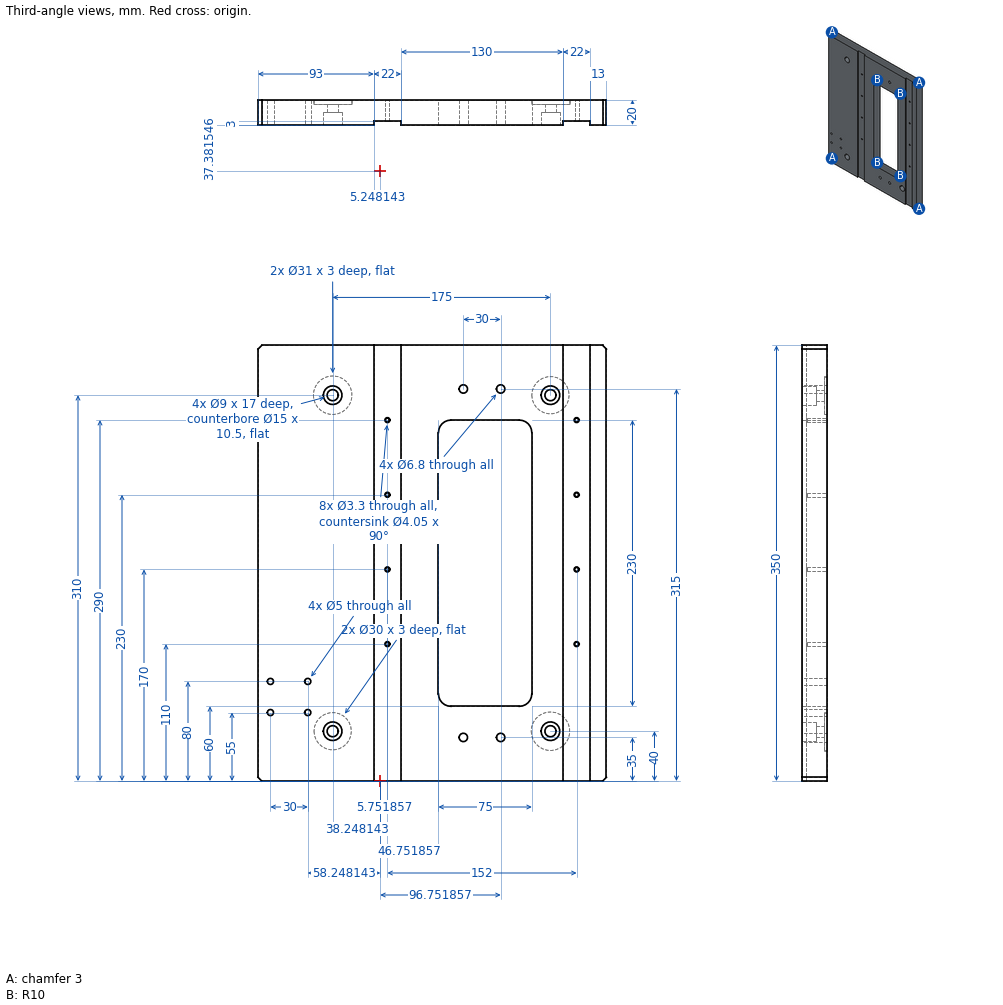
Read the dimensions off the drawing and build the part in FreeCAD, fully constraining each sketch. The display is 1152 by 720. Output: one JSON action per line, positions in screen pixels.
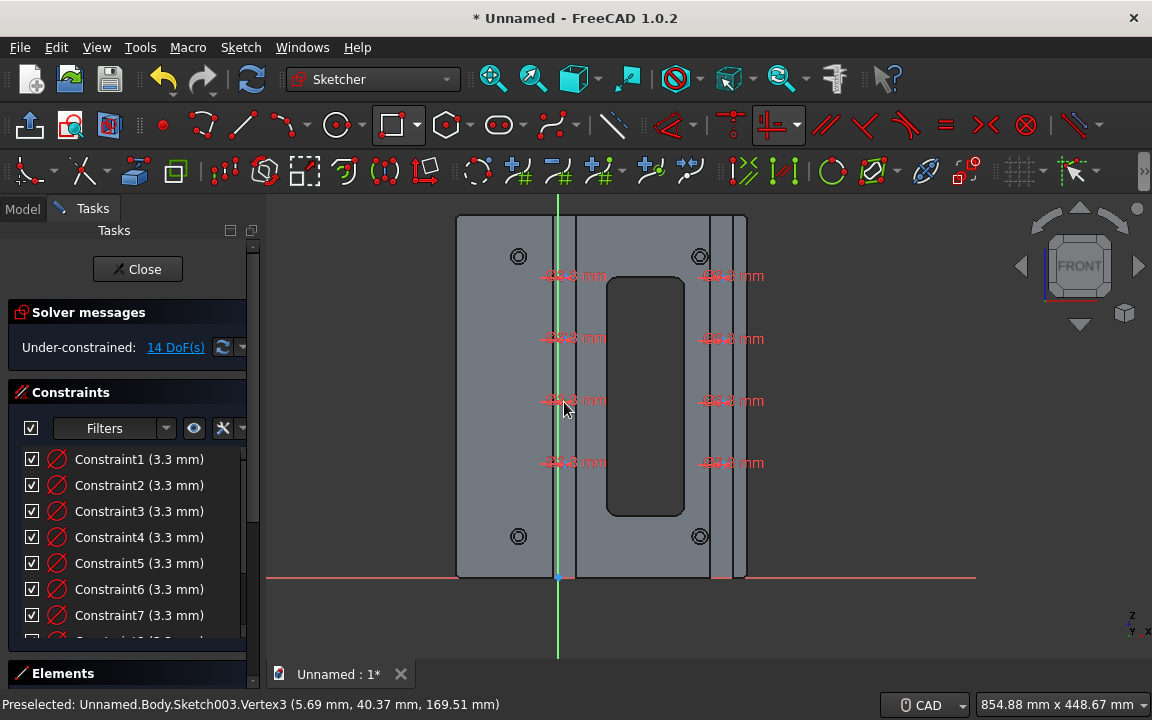
{"action": "left_click", "coordinate": [722, 403]}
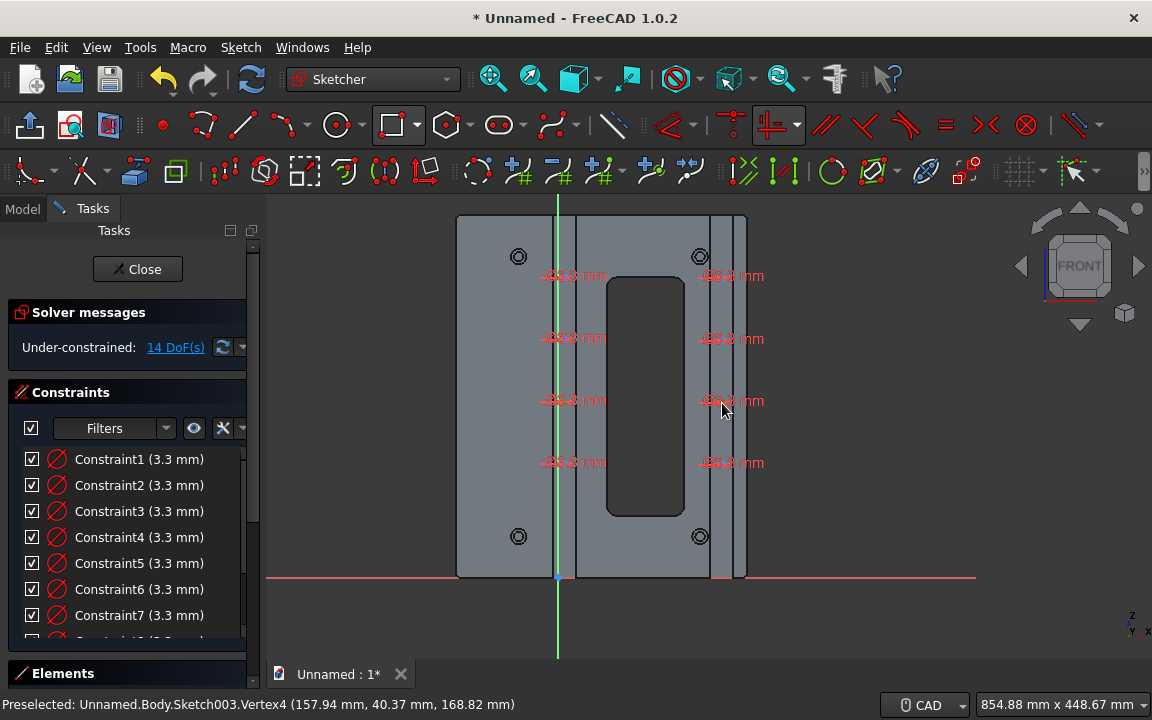
{"action": "key", "text": "h"}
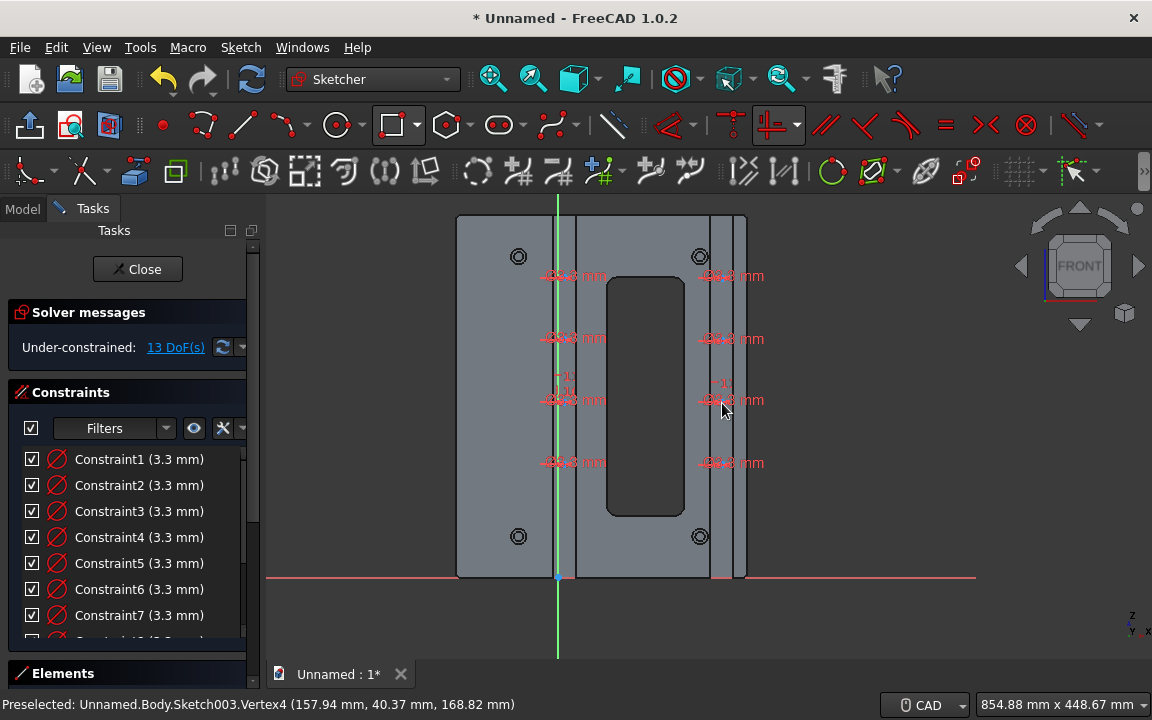
{"action": "left_click", "coordinate": [722, 402]}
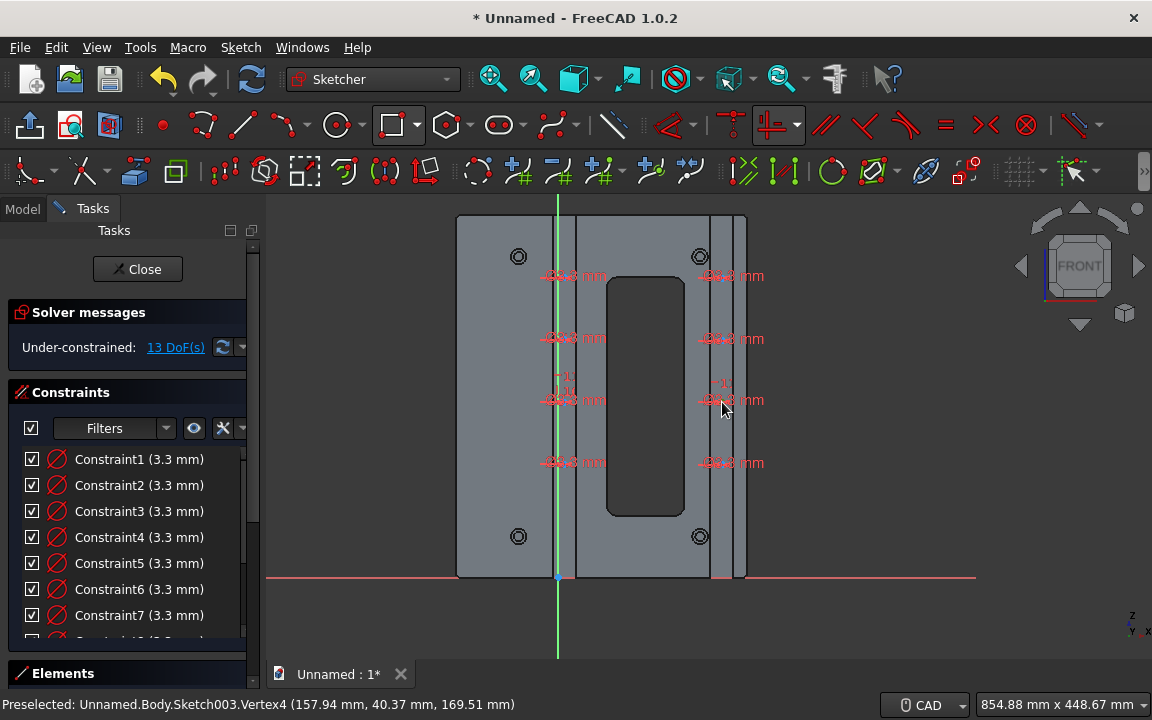
{"action": "left_click", "coordinate": [722, 341]}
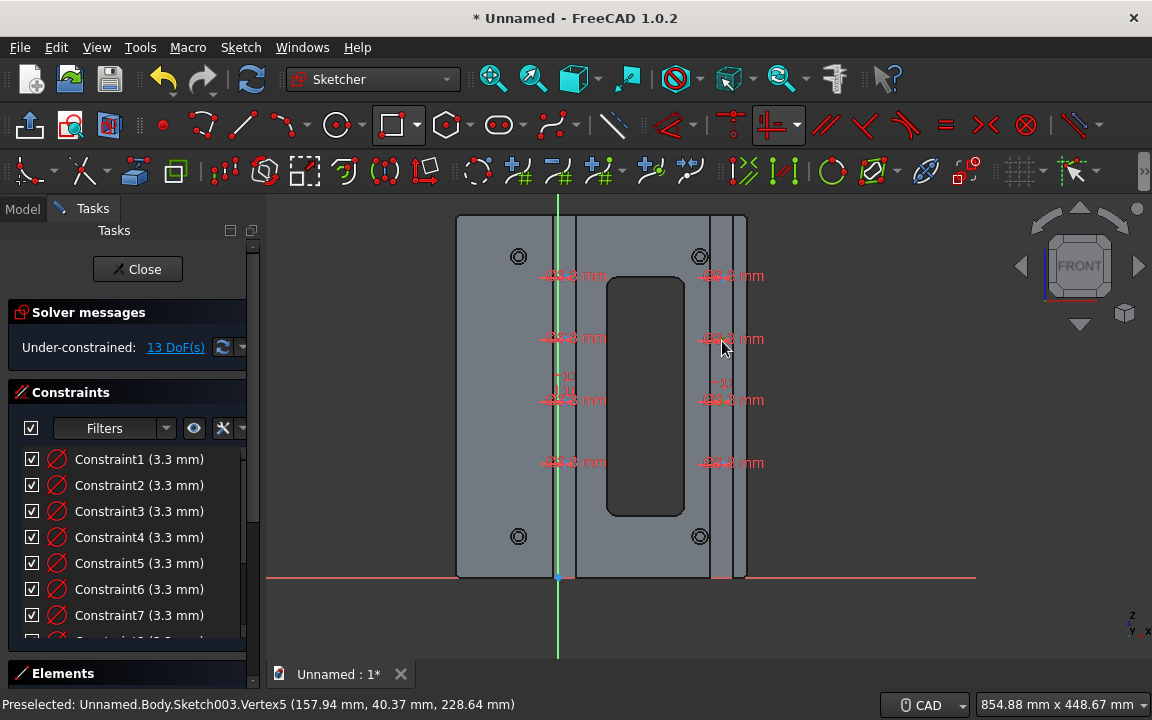
{"action": "key", "text": "v"}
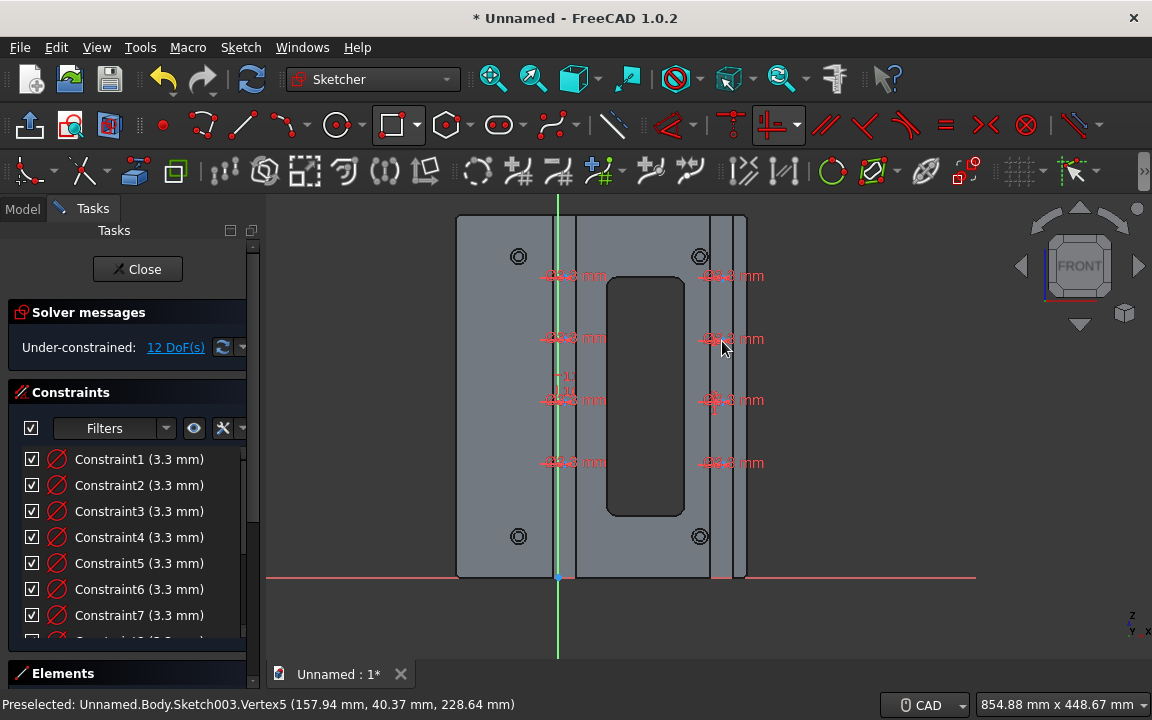
{"action": "left_click", "coordinate": [564, 340]}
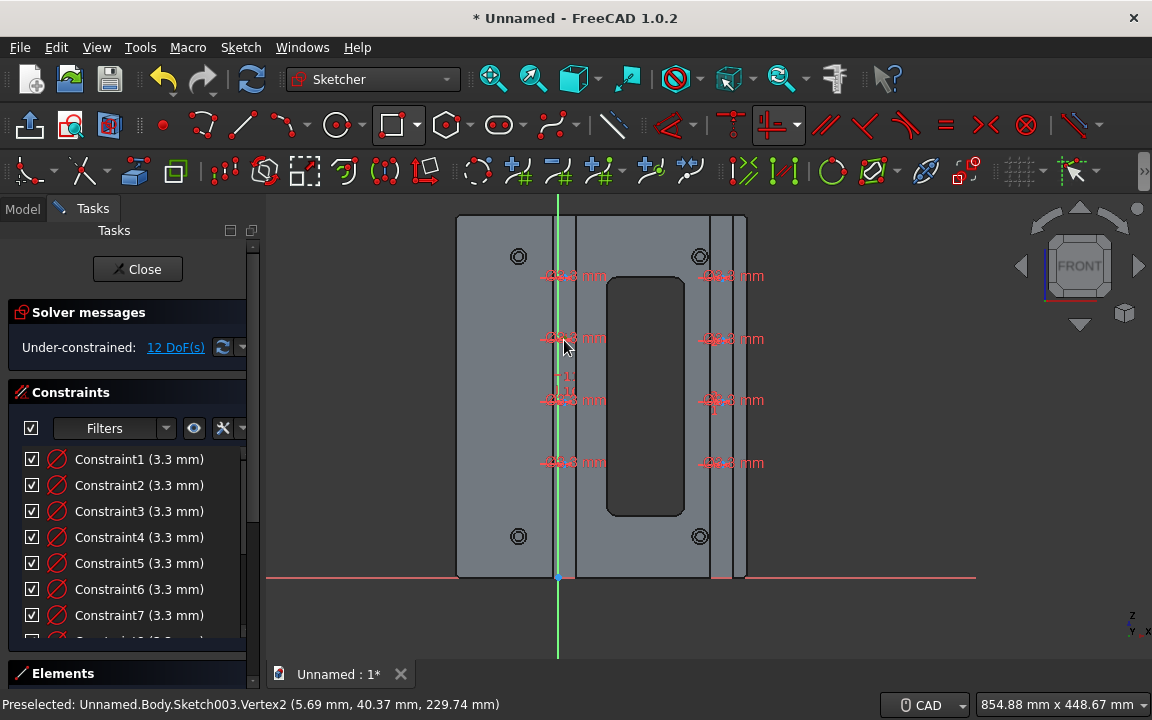
{"action": "left_click", "coordinate": [722, 341]}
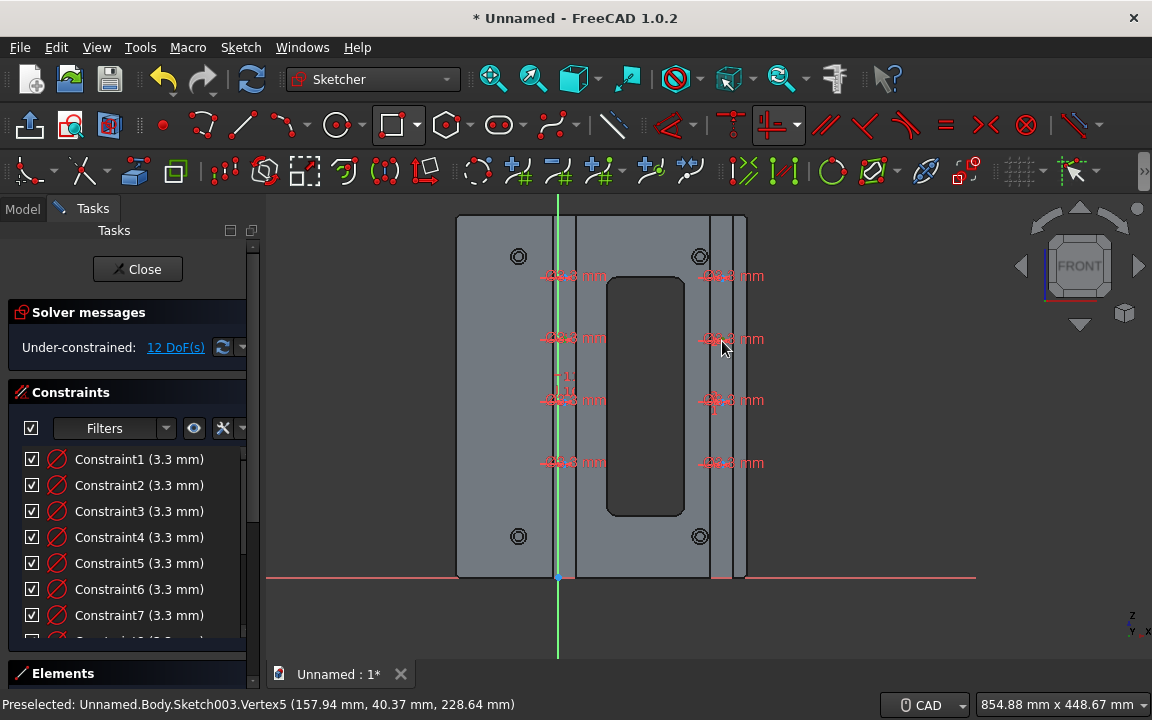
{"action": "left_click", "coordinate": [800, 126]}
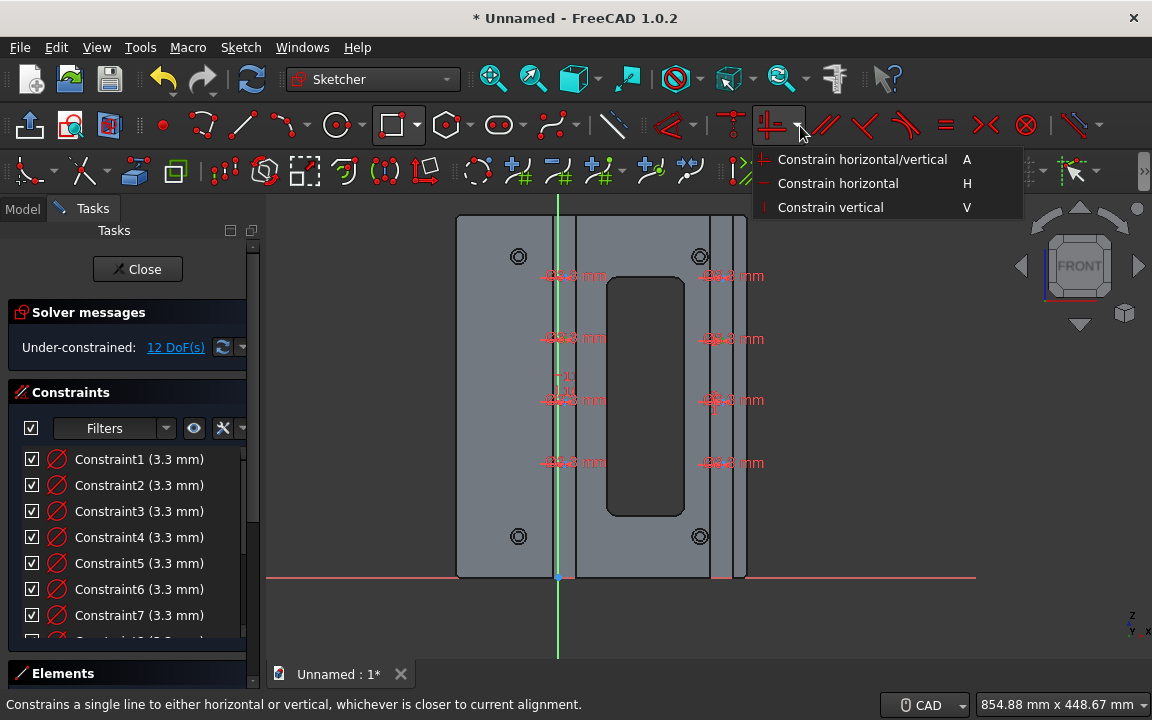
{"action": "left_click", "coordinate": [888, 183]}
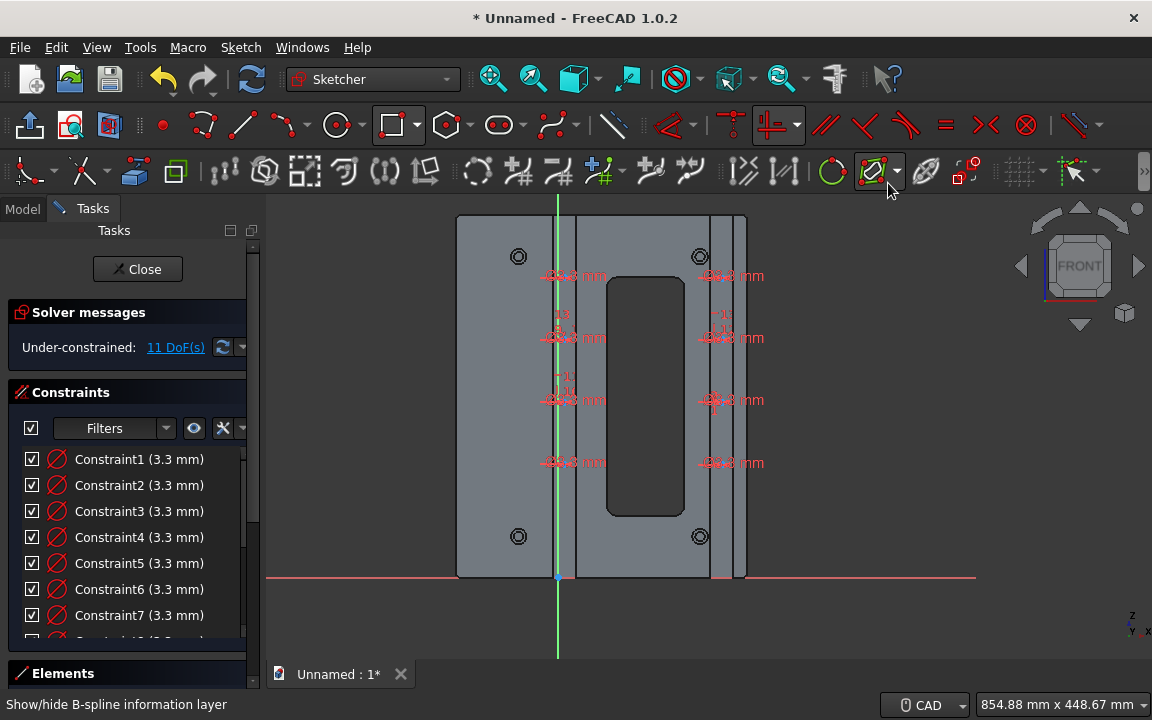
{"action": "left_click", "coordinate": [722, 340]}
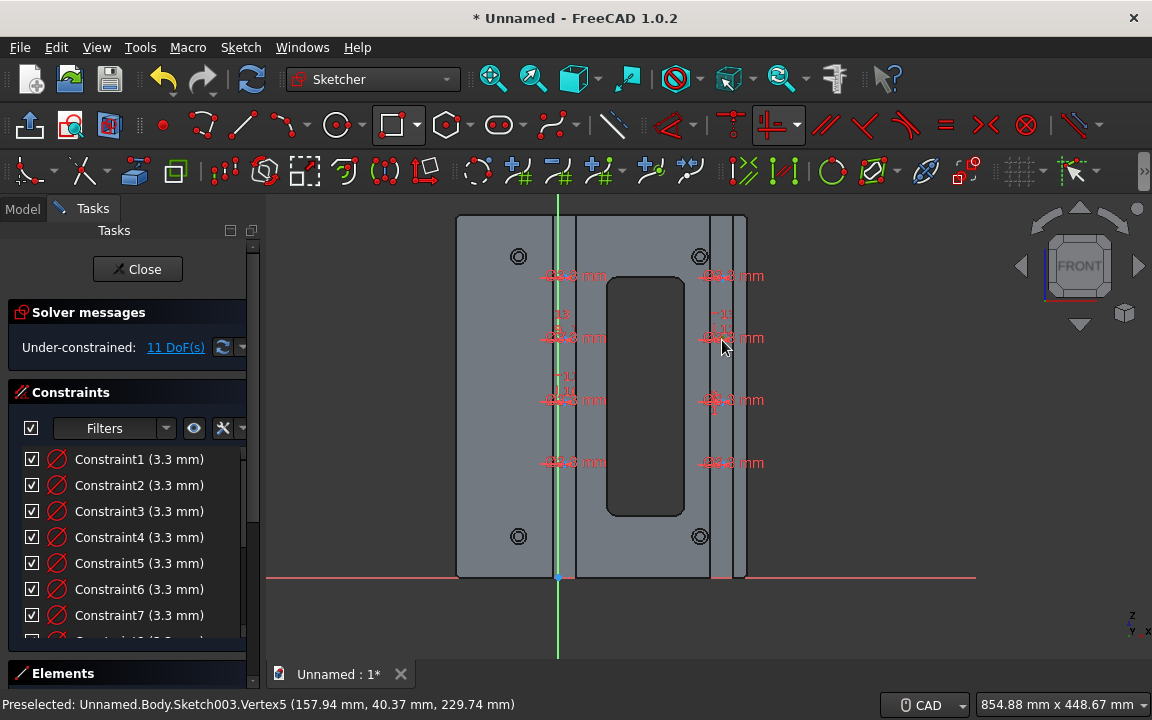
{"action": "left_click", "coordinate": [722, 278]}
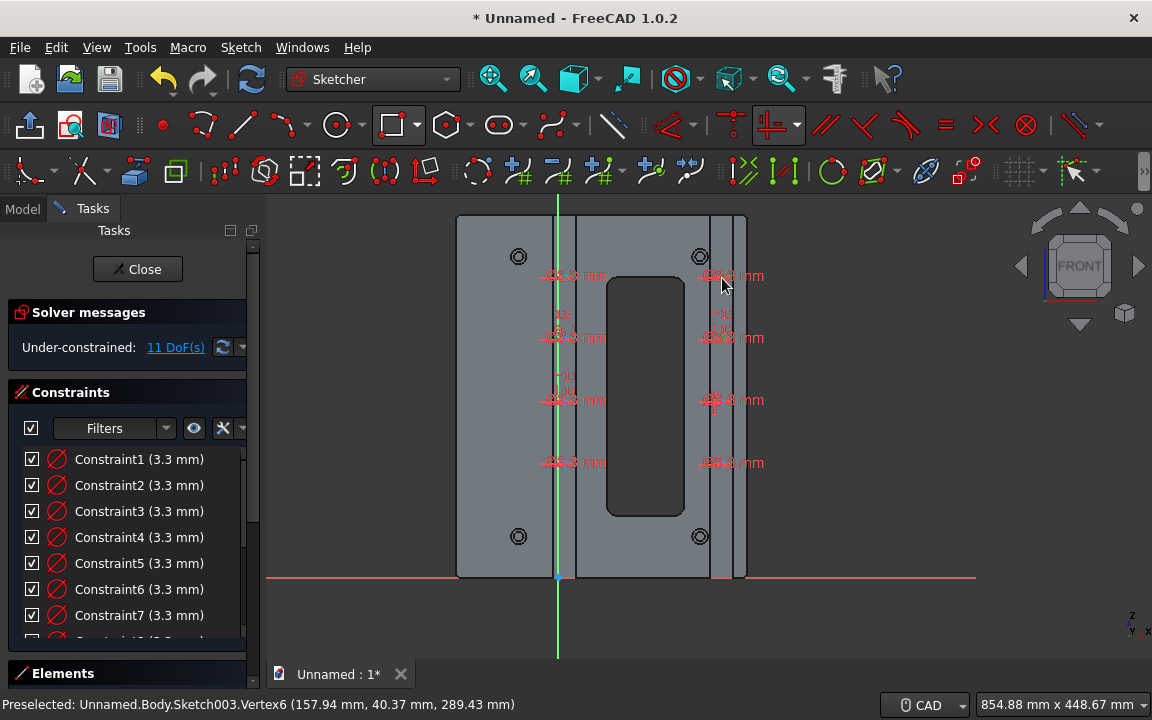
{"action": "key", "text": "v"}